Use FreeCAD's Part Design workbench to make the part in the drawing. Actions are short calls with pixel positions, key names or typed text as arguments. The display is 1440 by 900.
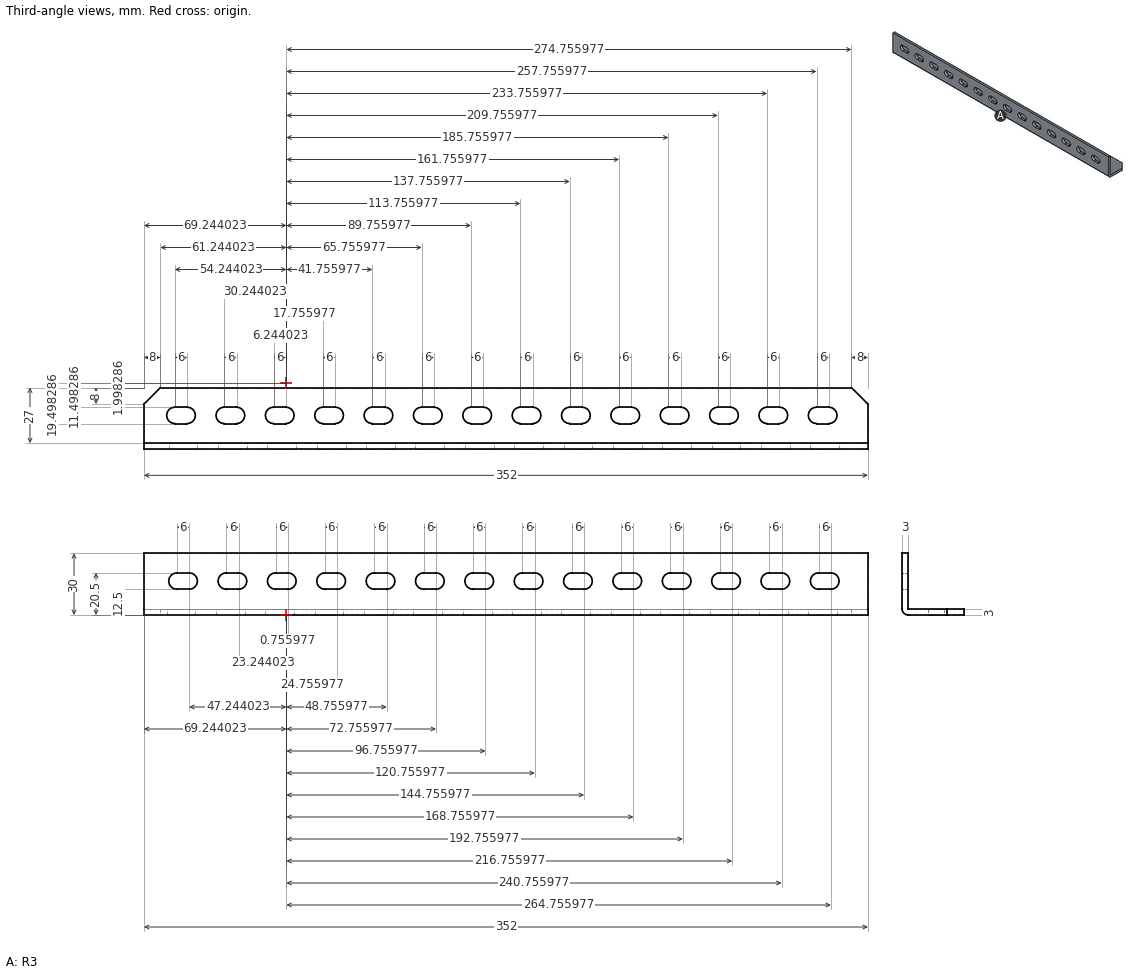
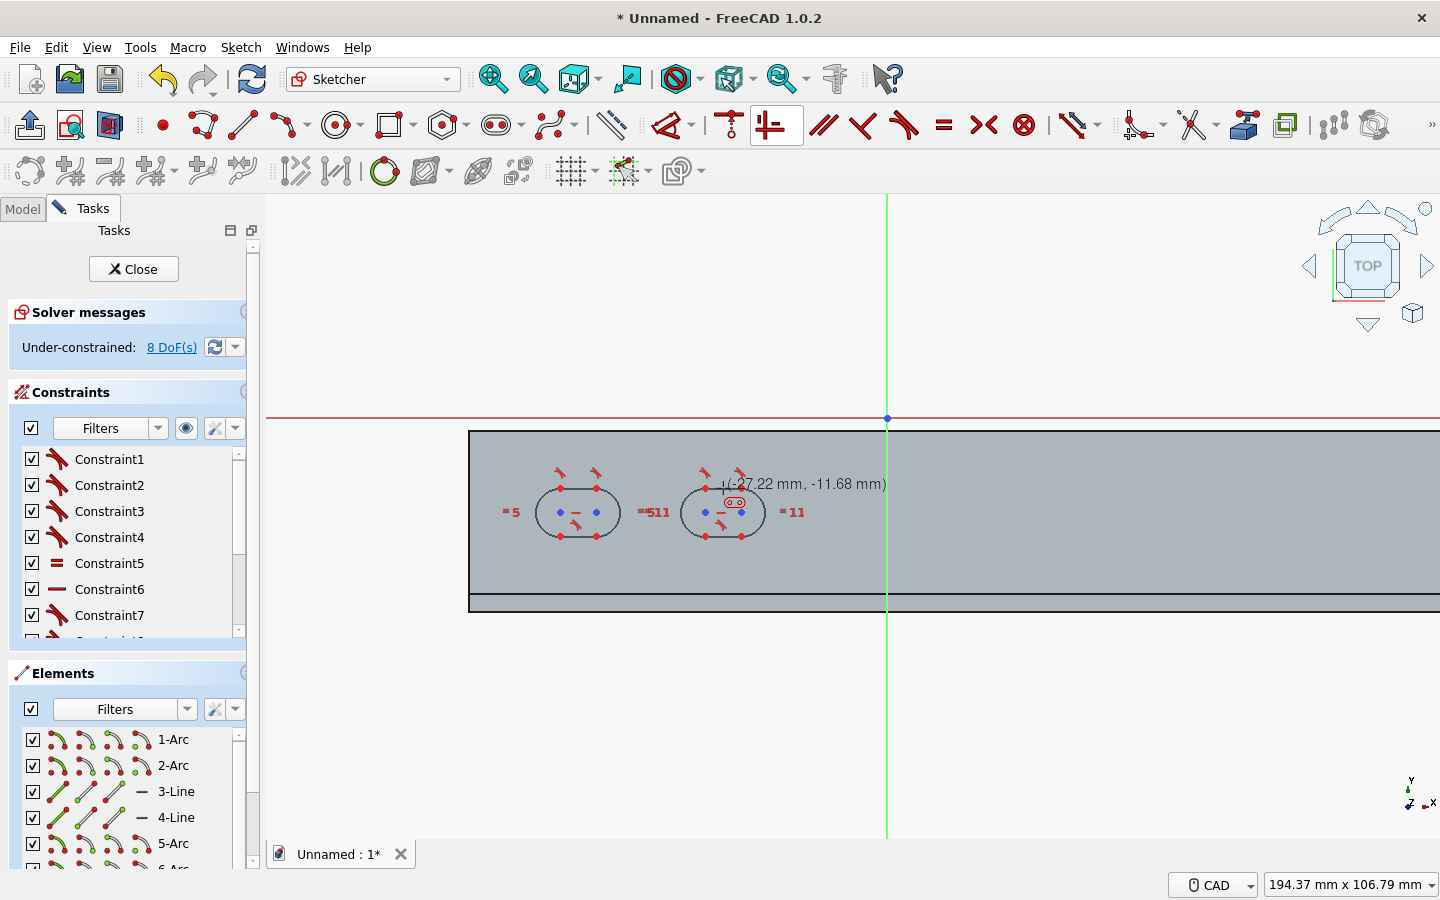
click(850, 512)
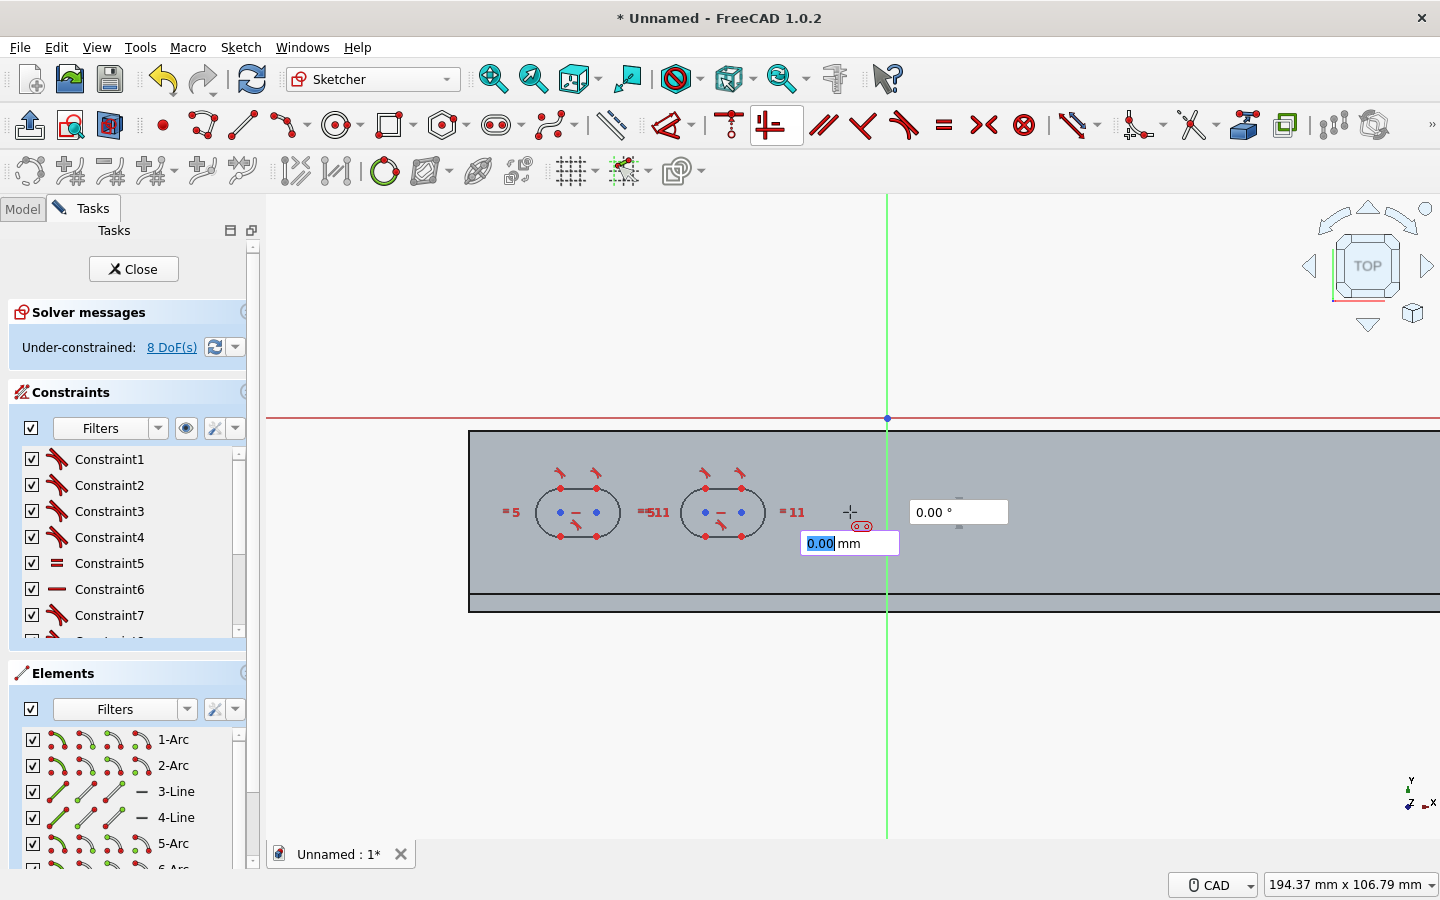
scroll(886, 512, up, 12)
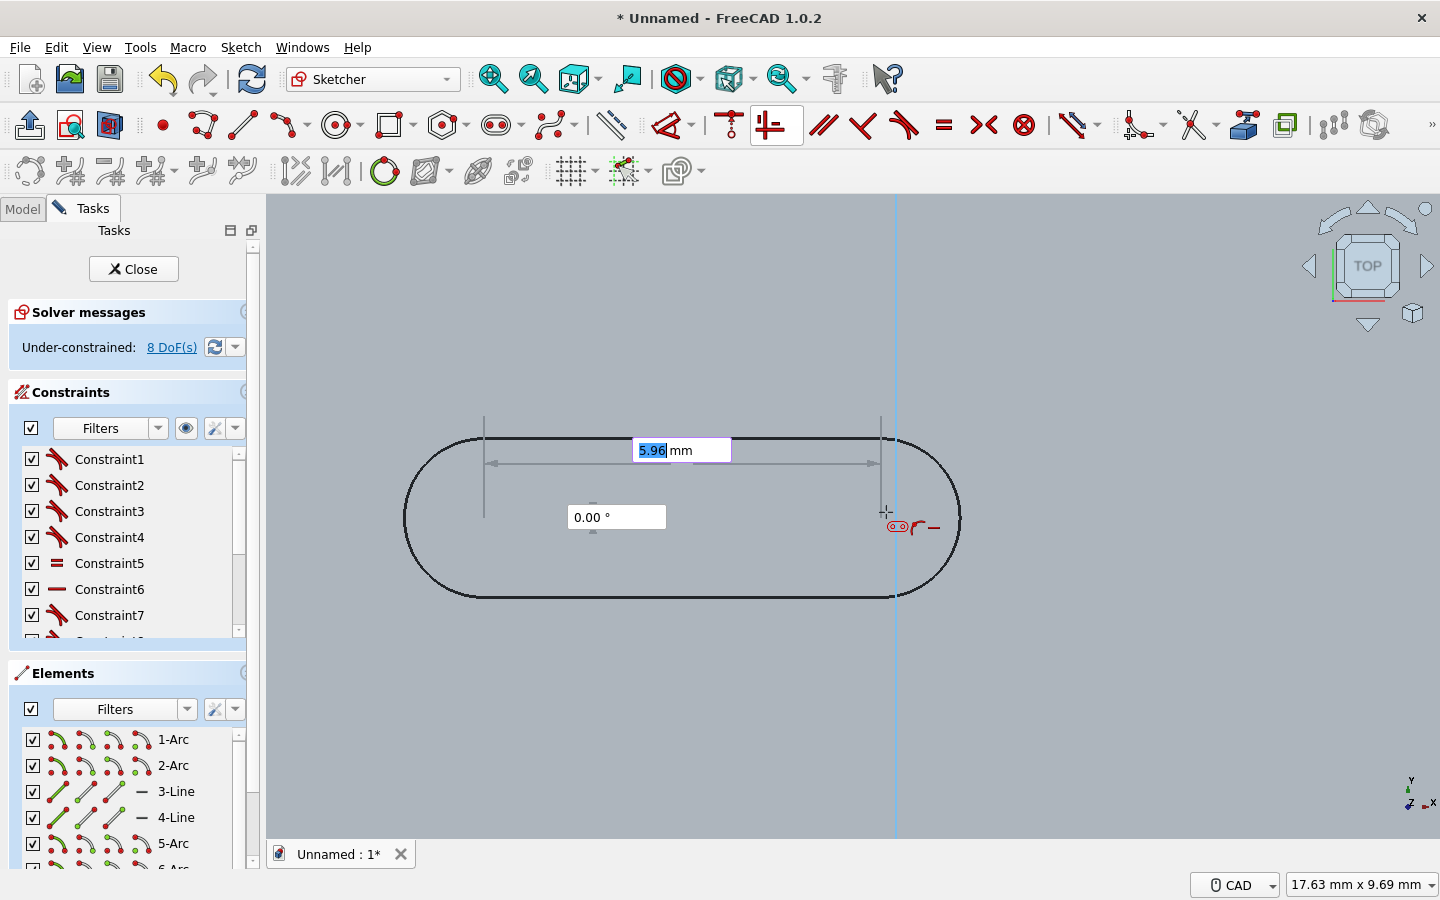
click(880, 507)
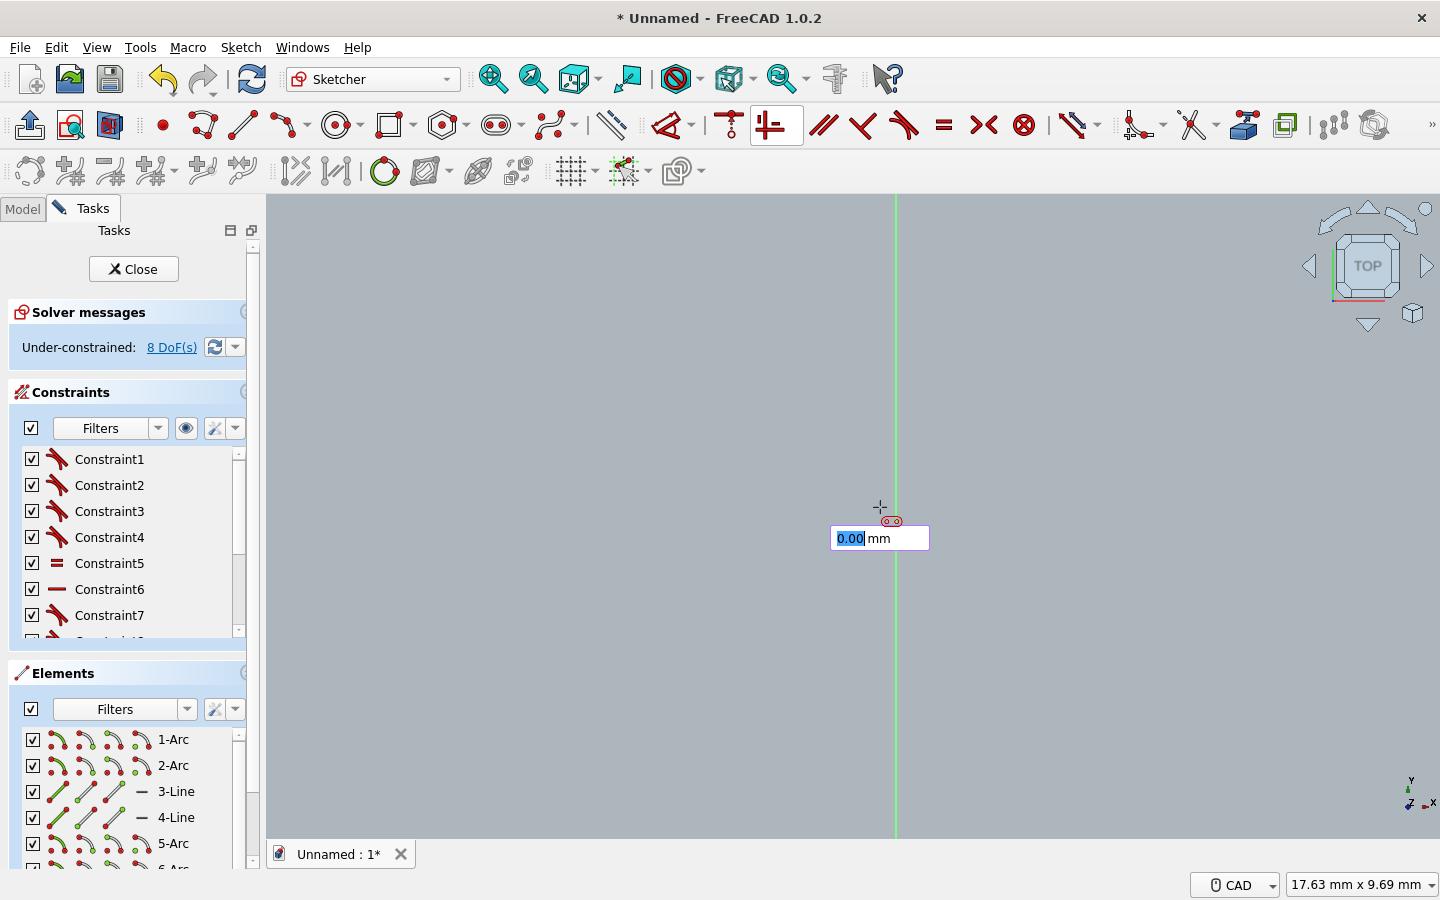
scroll(483, 533, down, 16)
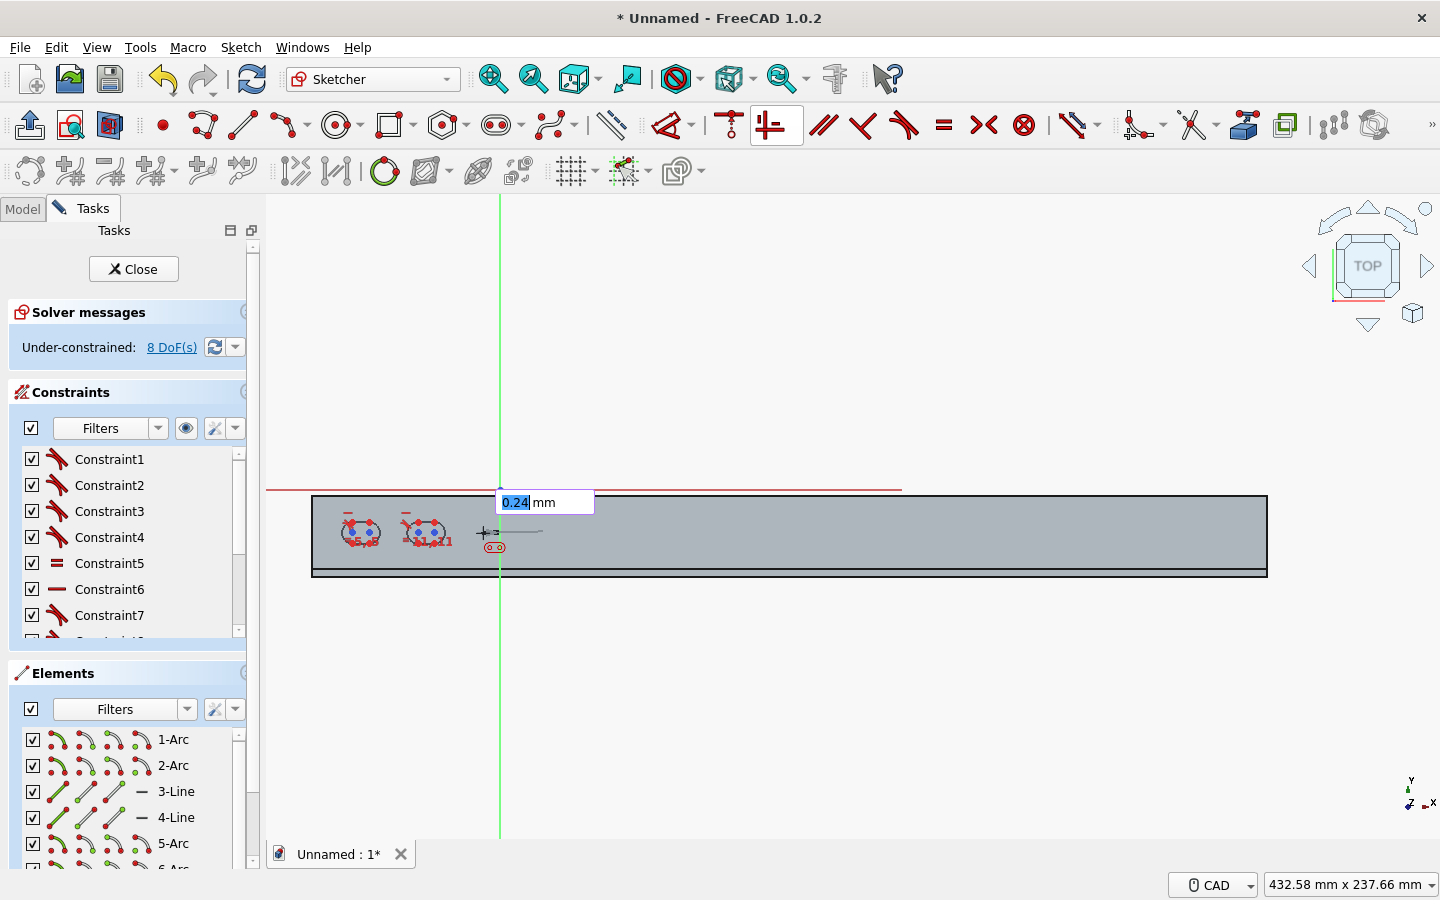
scroll(491, 522, up, 3)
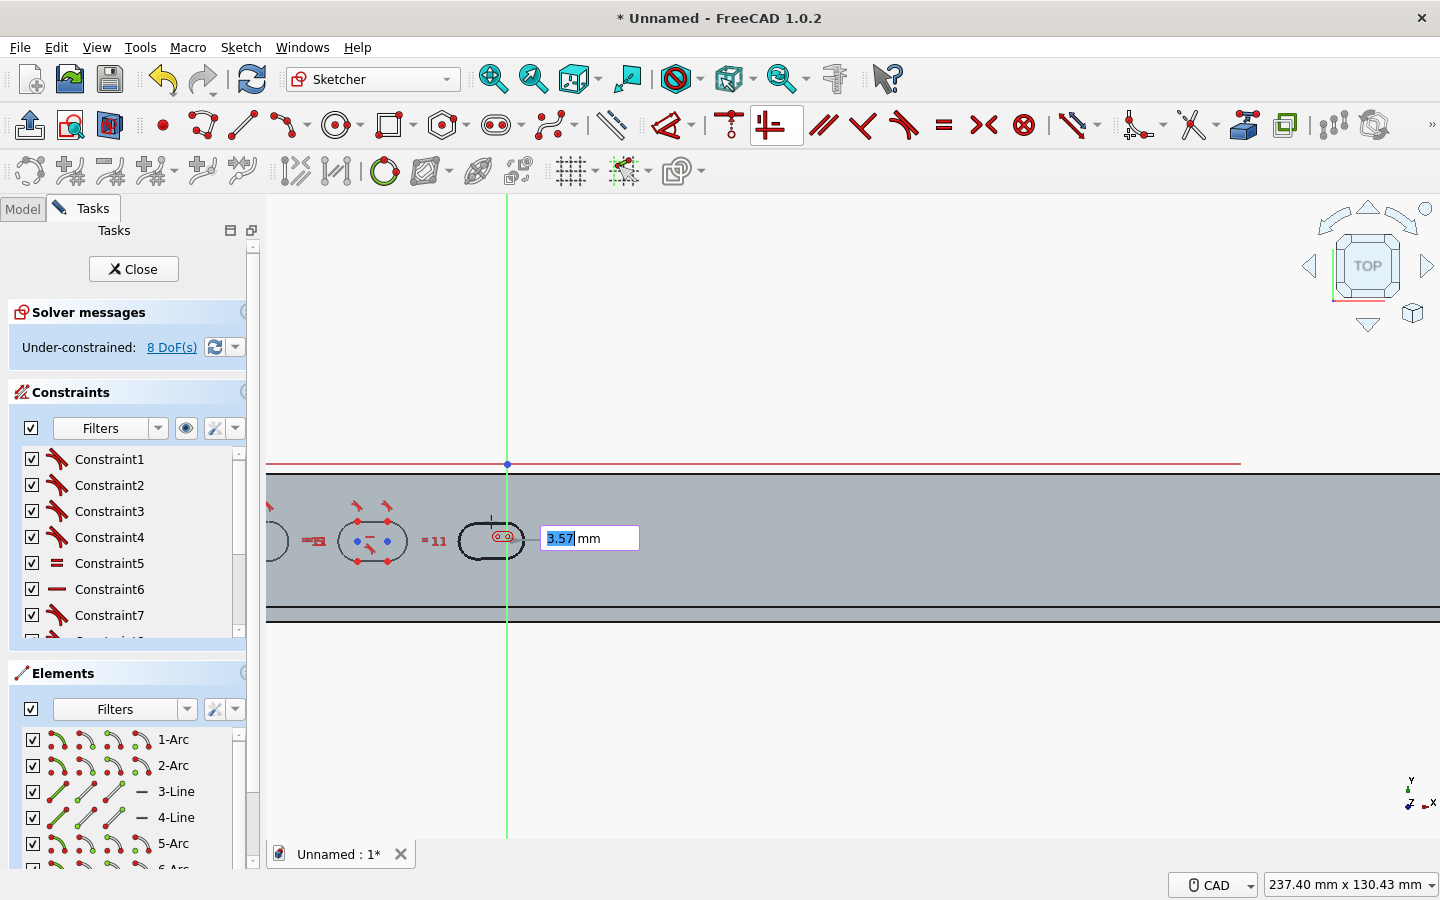
click(491, 521)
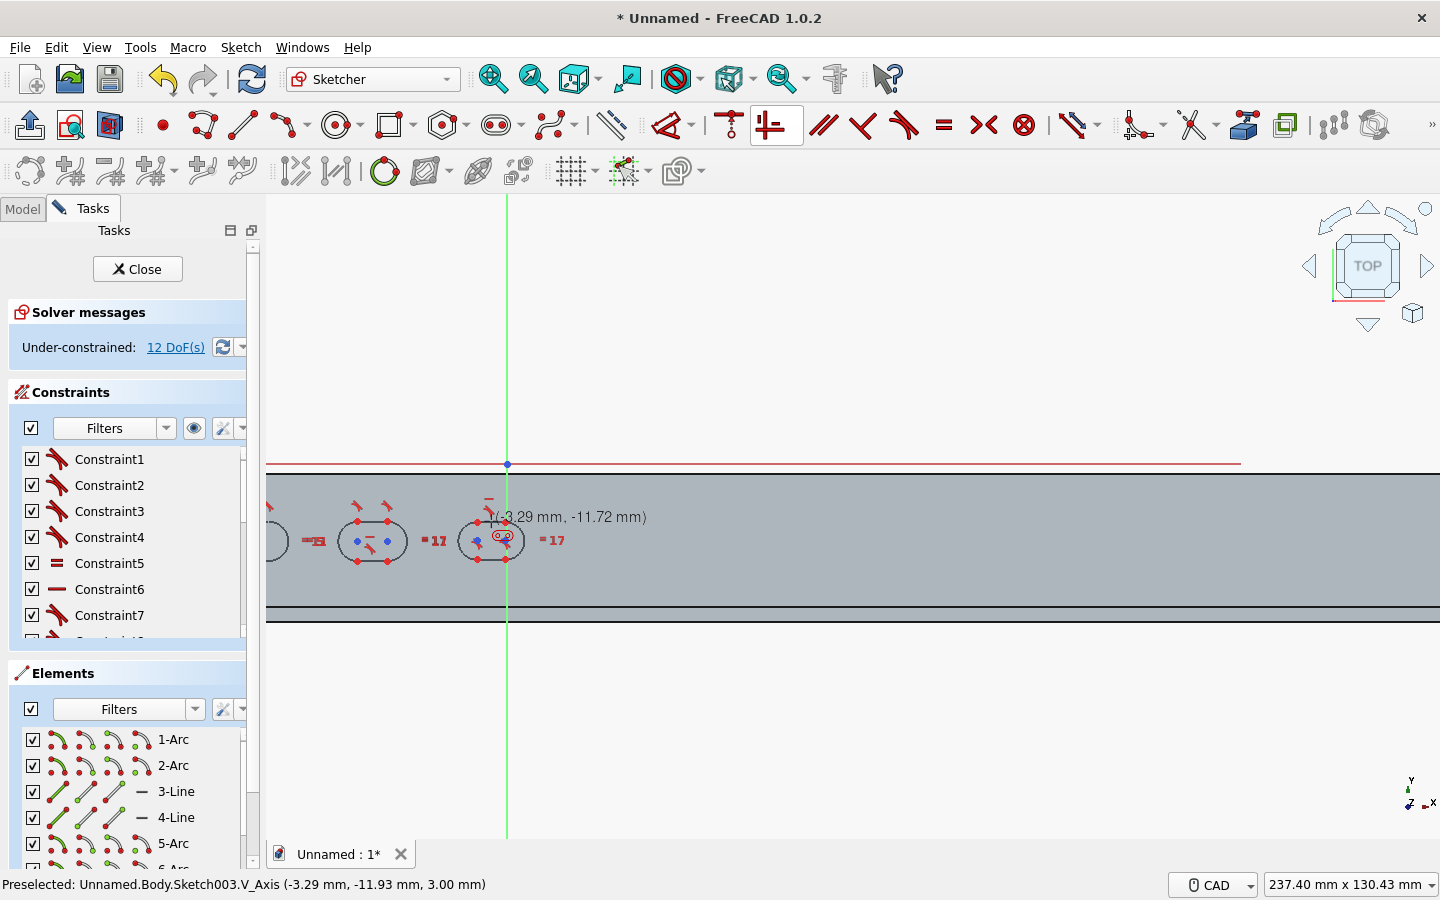
click(595, 541)